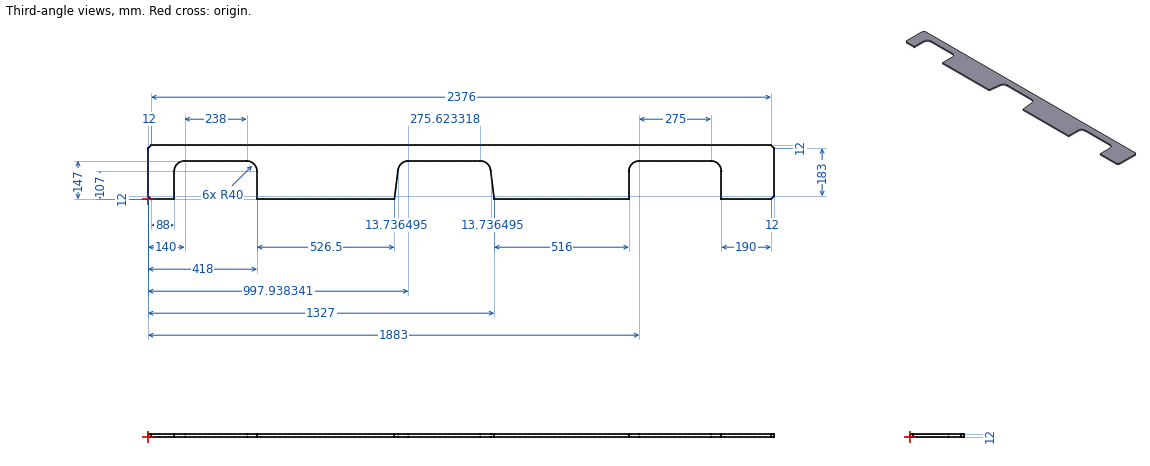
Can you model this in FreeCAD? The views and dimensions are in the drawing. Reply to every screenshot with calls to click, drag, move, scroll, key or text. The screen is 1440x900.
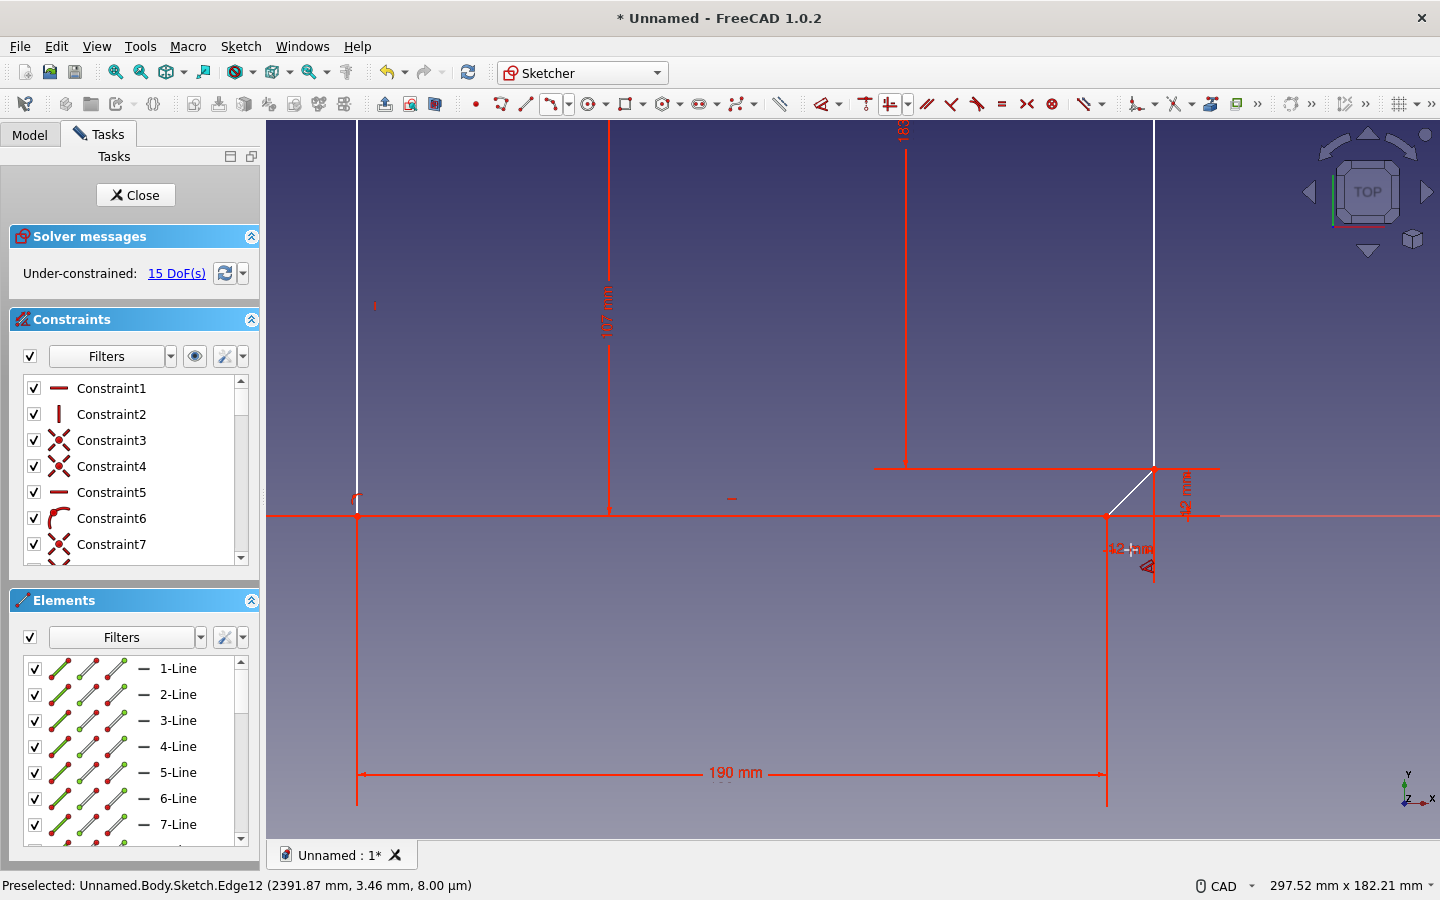
scroll(1135, 509, down, 13)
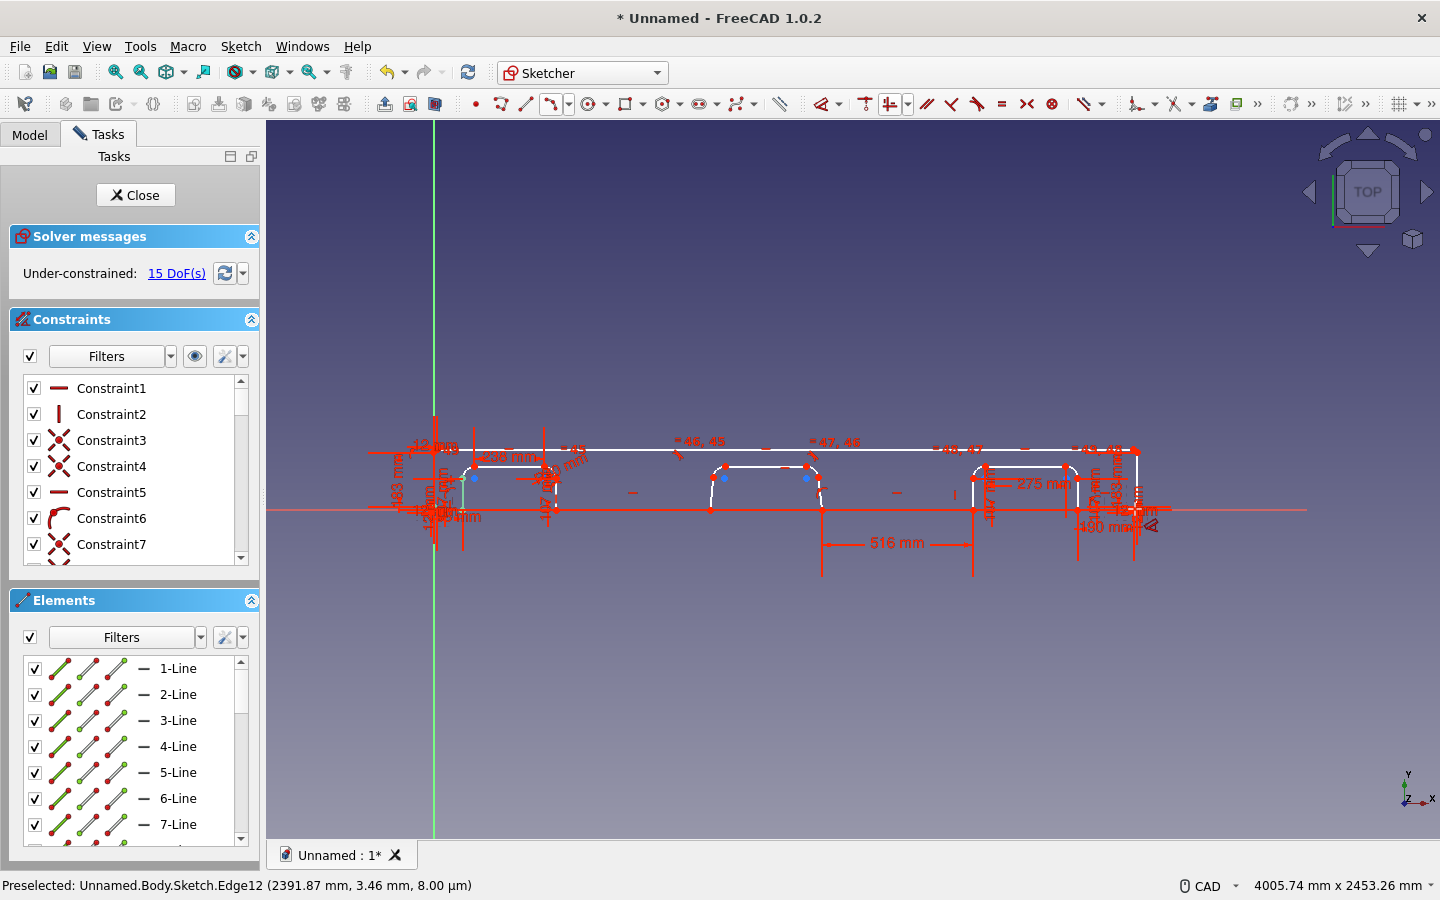
scroll(1136, 452, up, 13)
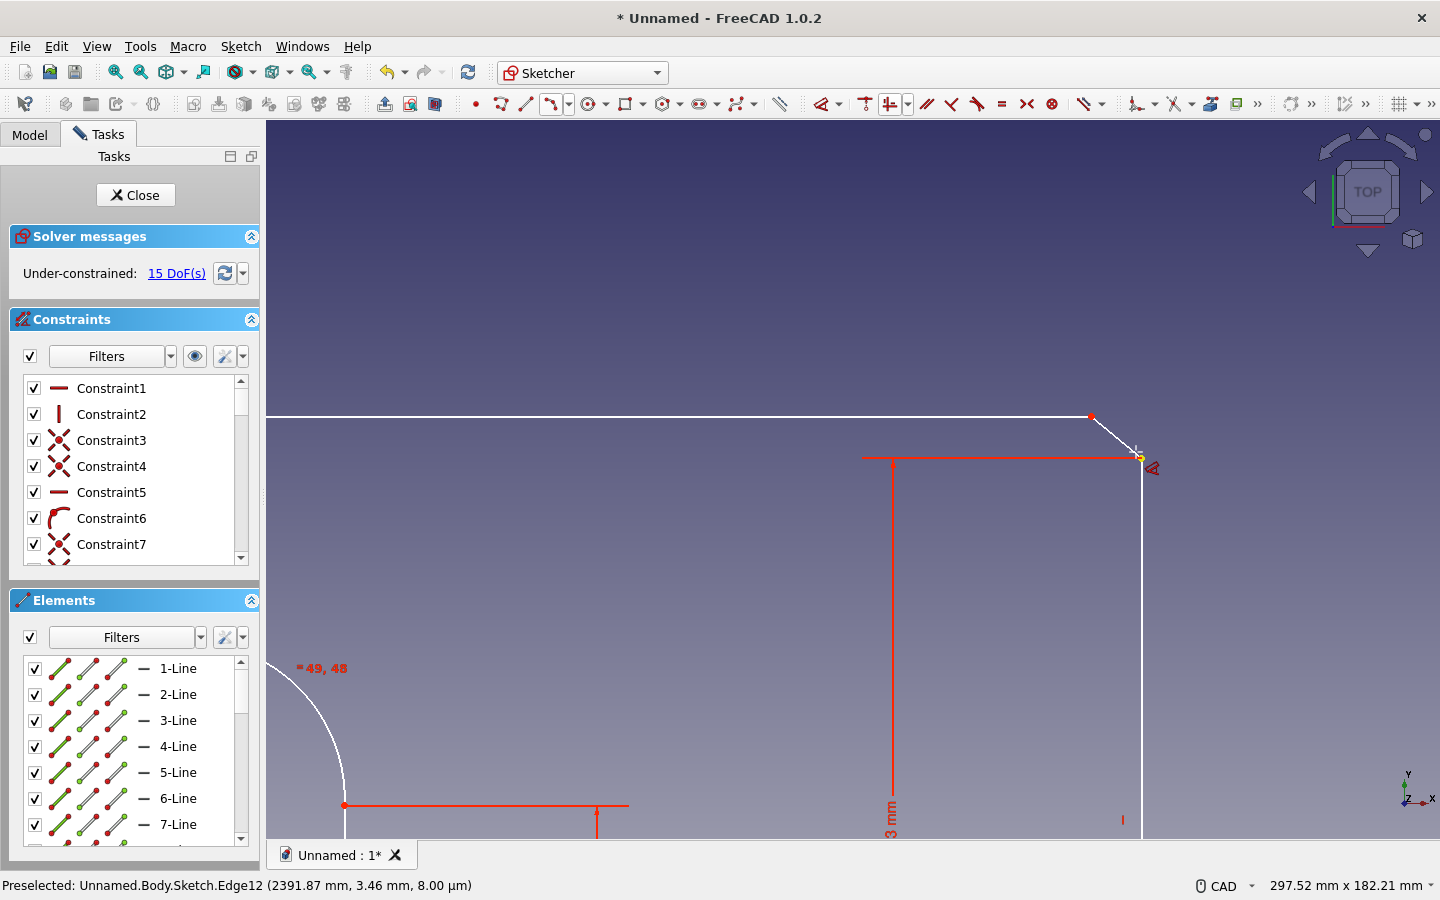
click(1127, 446)
click(1116, 383)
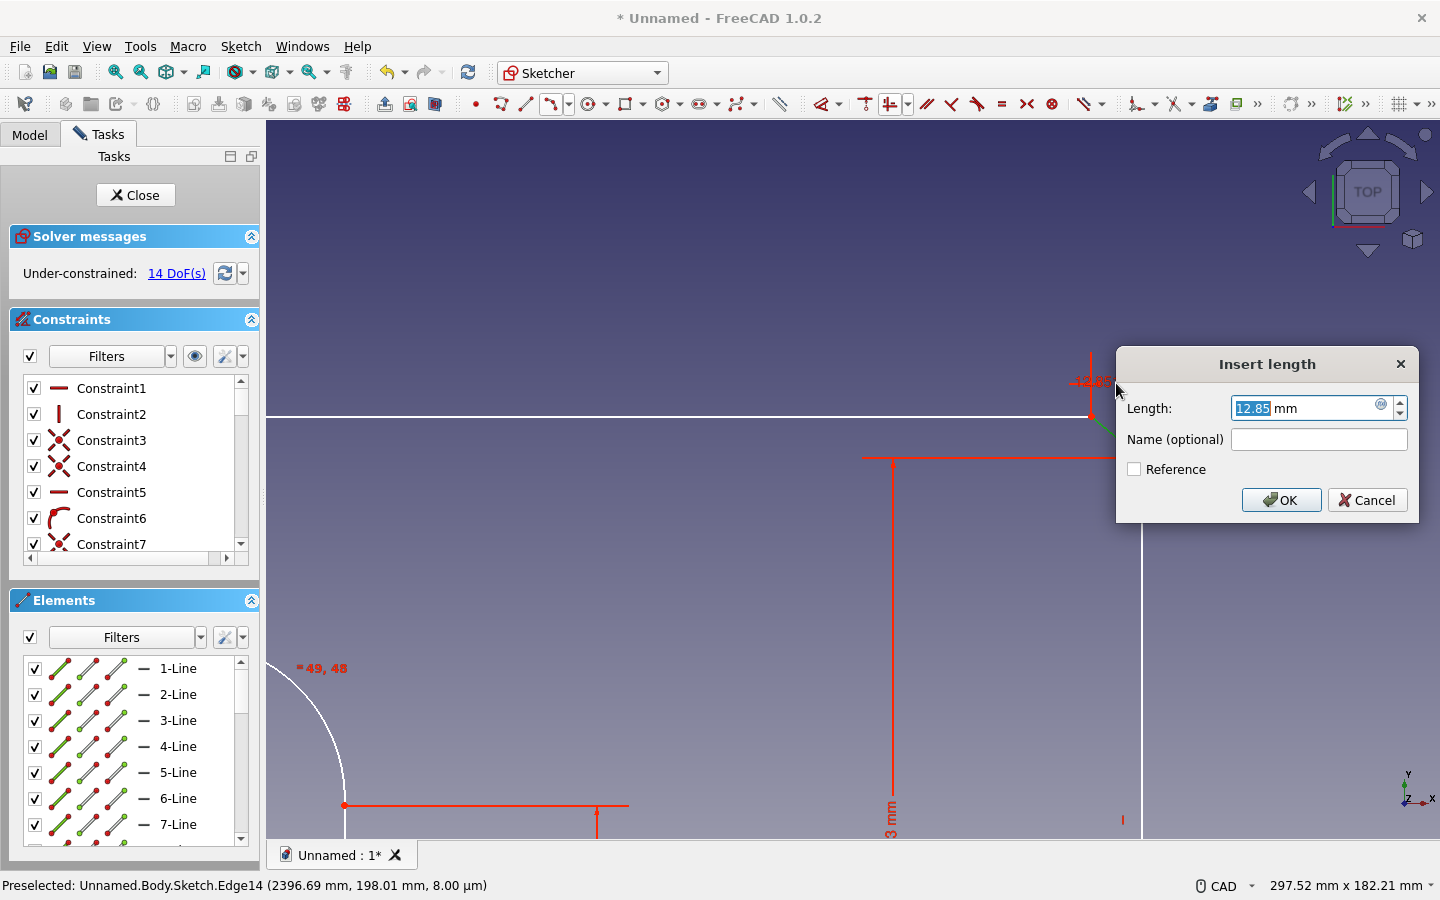
text(12)
key(Return)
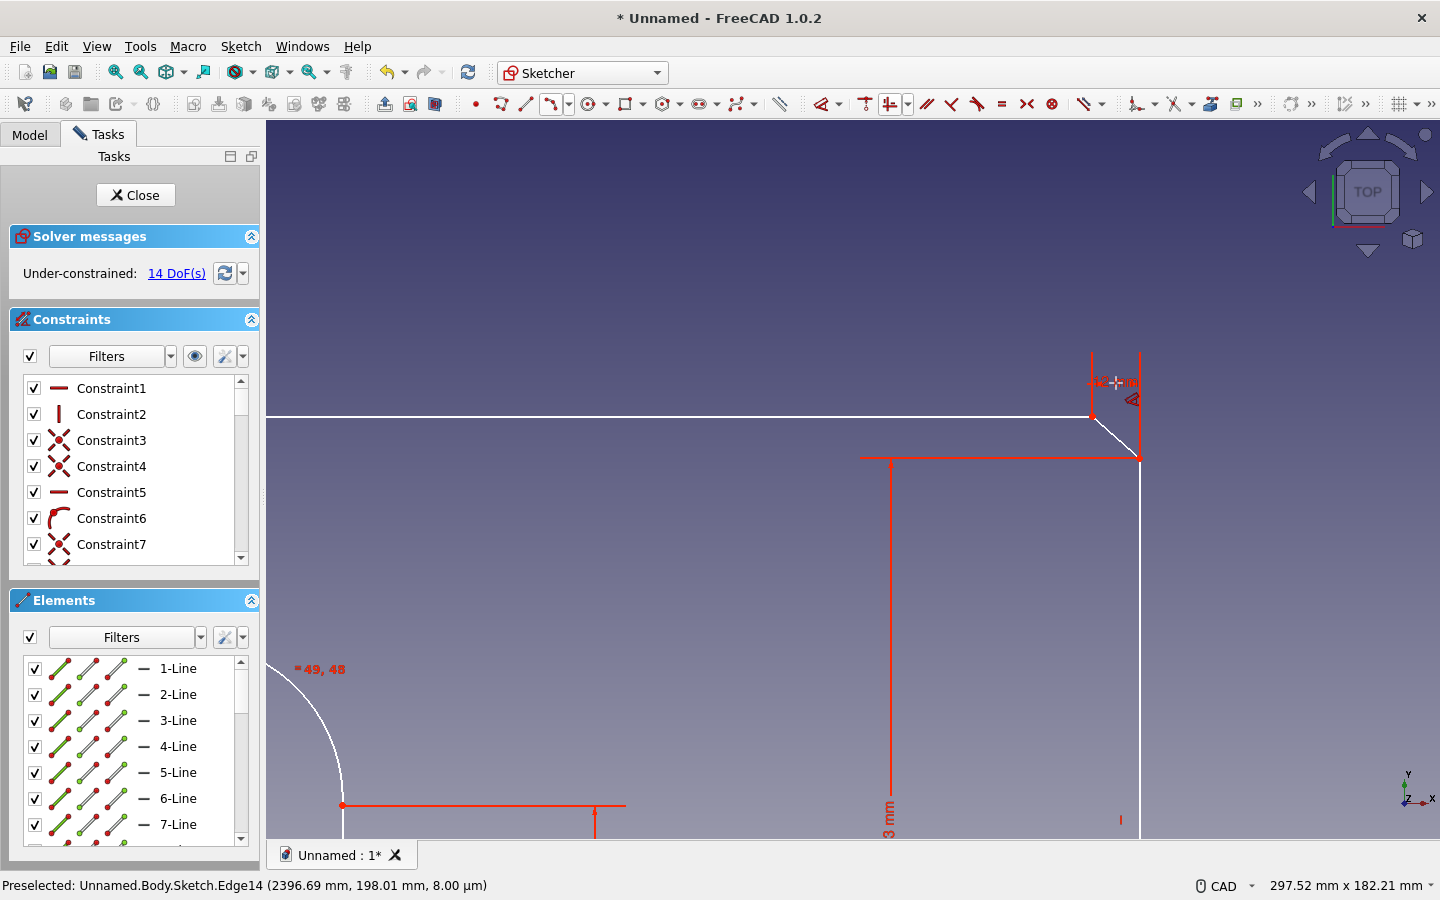
click(1125, 446)
click(1174, 438)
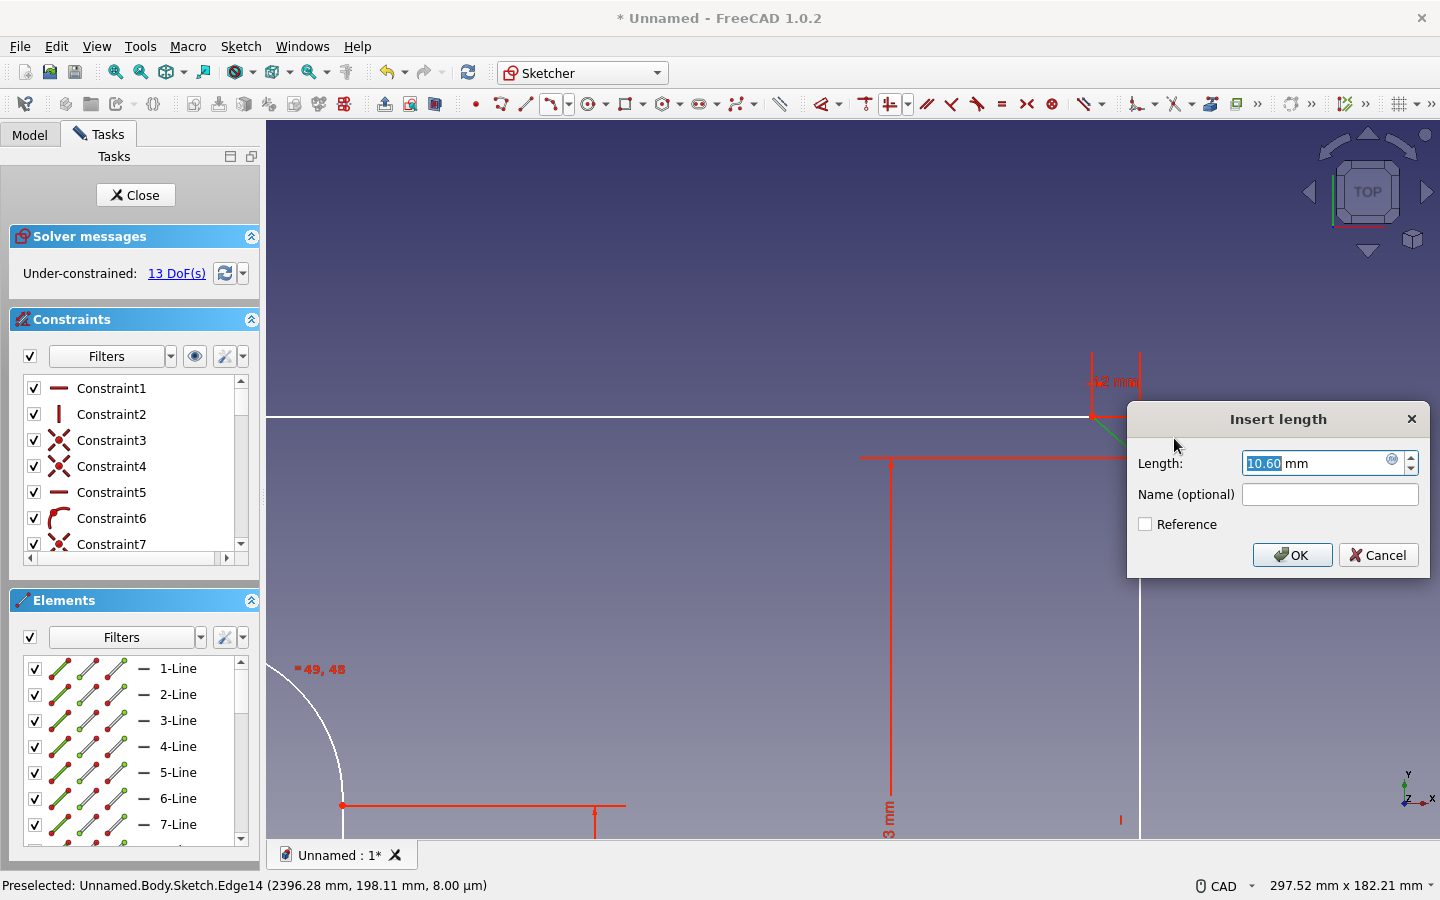
text(12)
key(Return)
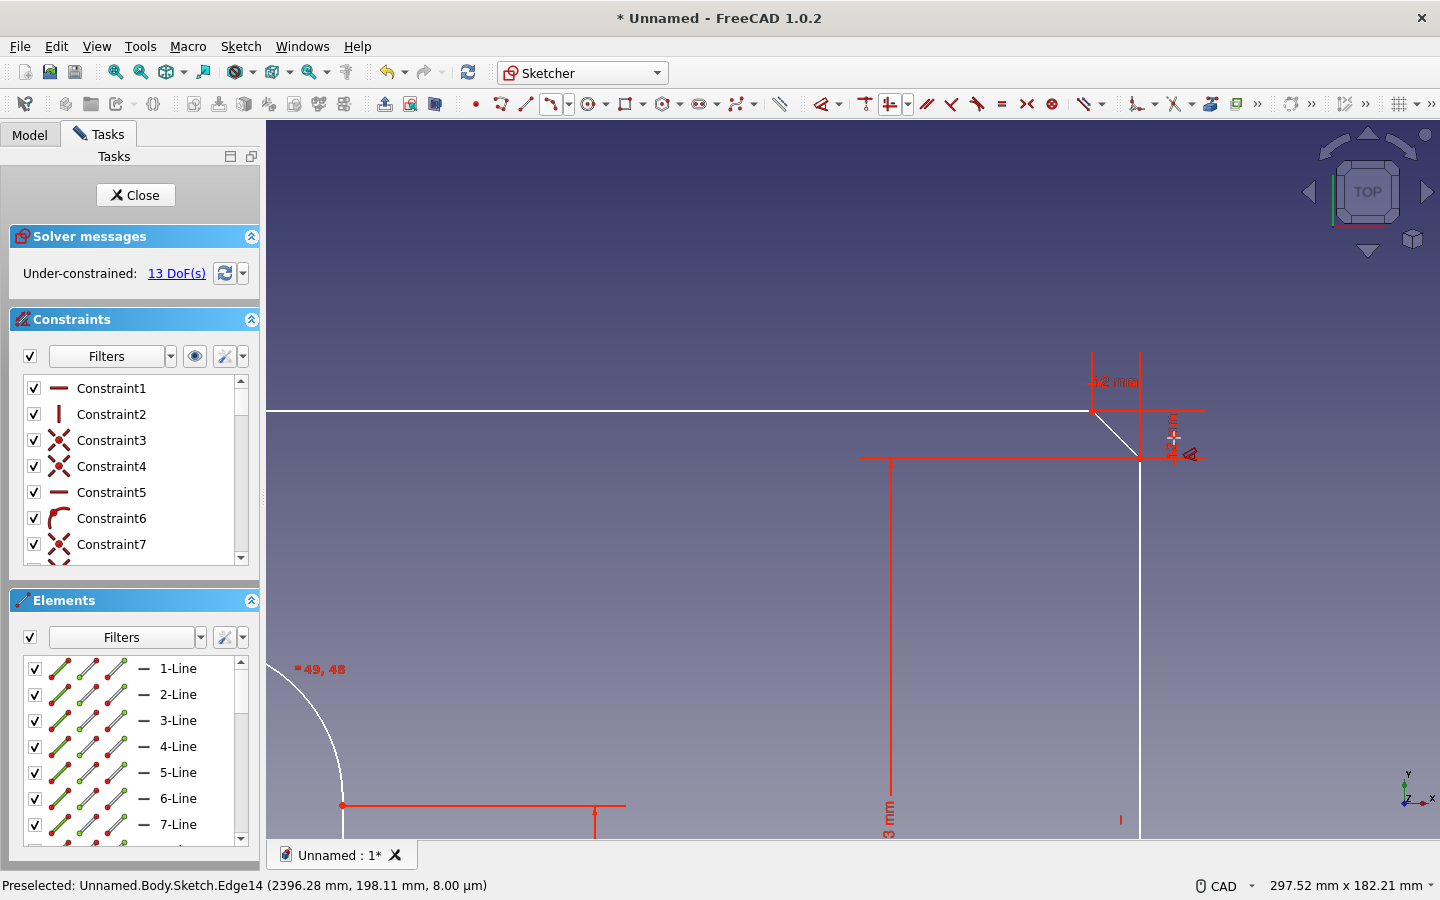
scroll(1136, 452, down, 13)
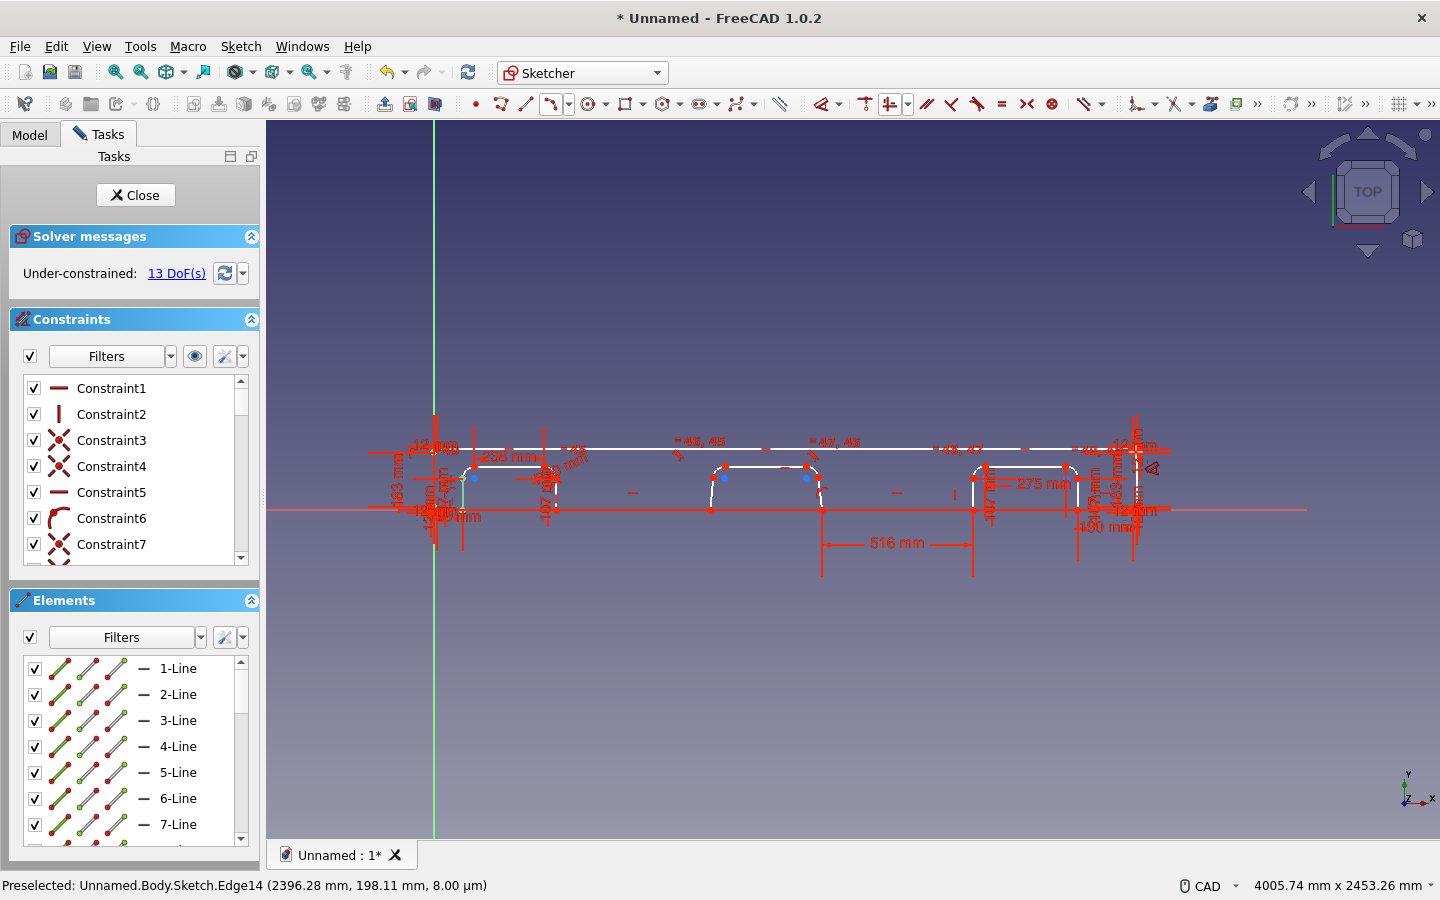
click(925, 449)
click(785, 415)